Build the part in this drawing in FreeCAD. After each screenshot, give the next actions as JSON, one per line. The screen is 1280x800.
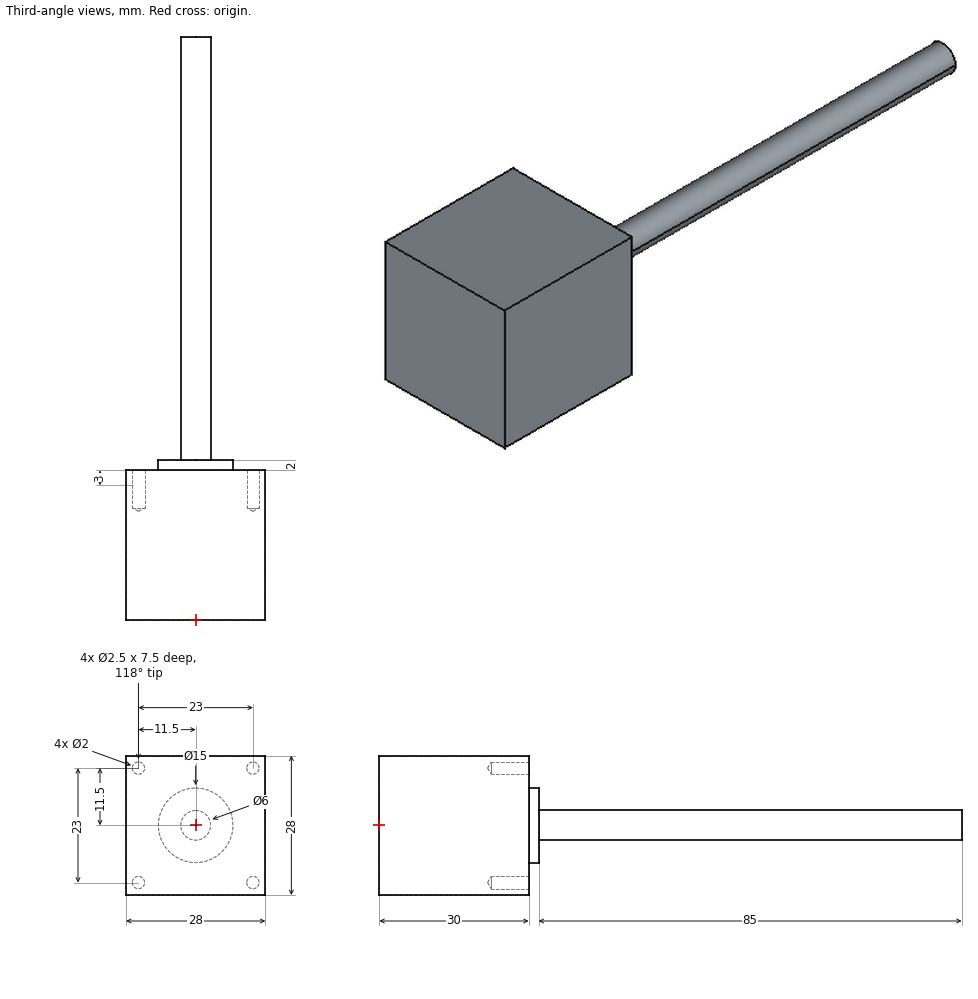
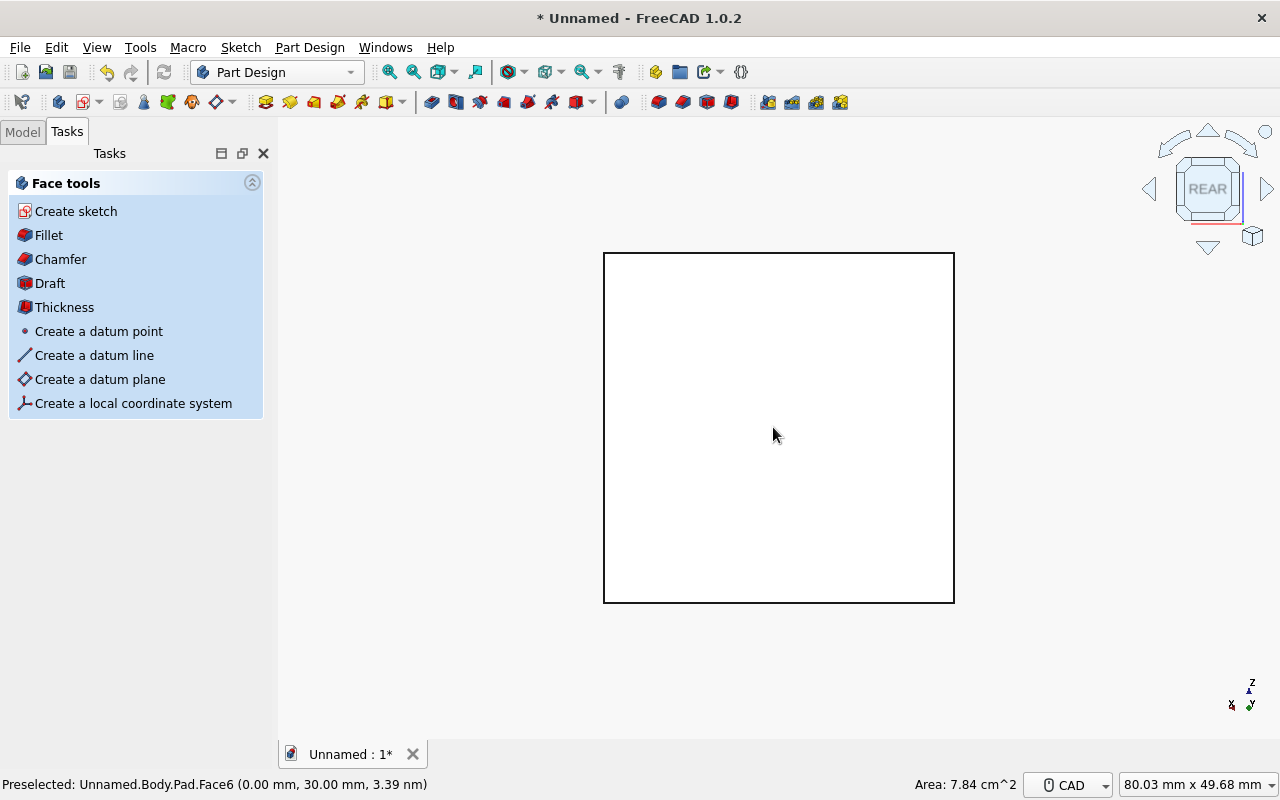
{"action": "left_click", "coordinate": [84, 102]}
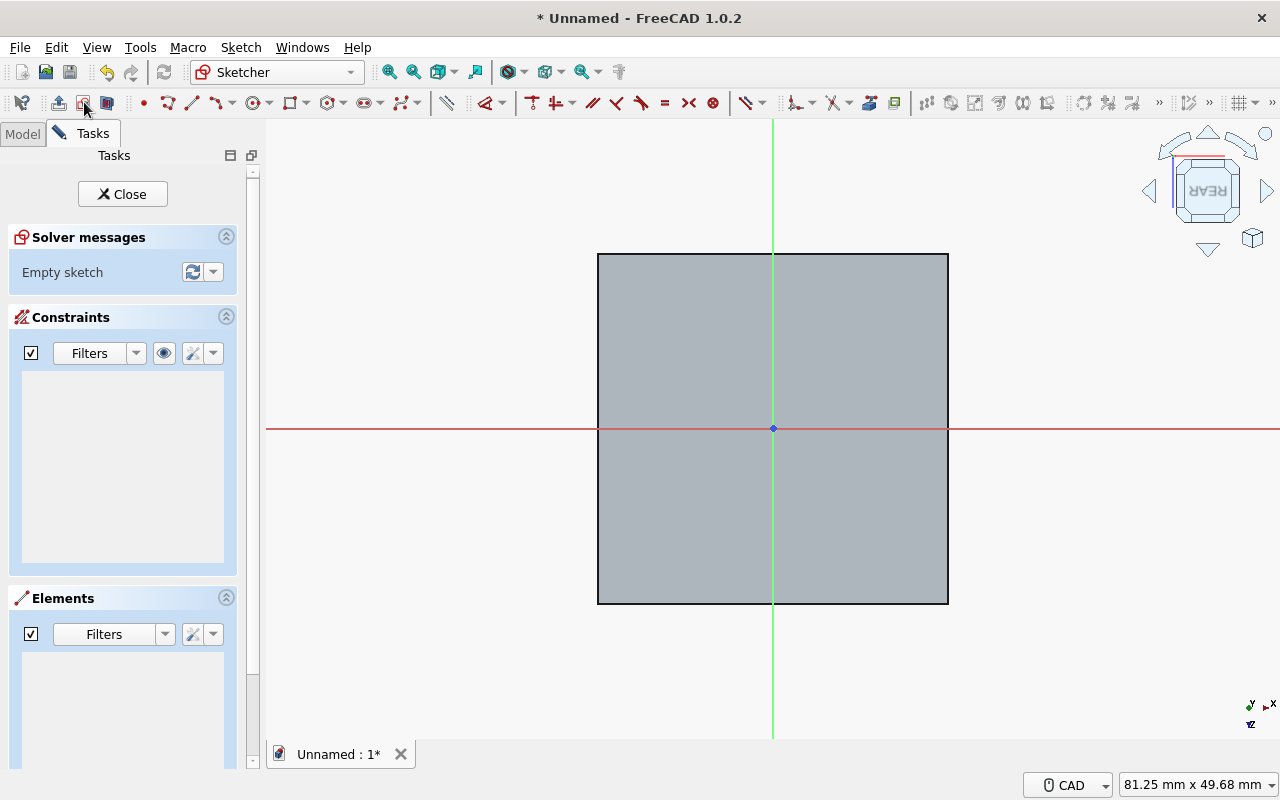
{"action": "scroll", "coordinate": [829, 429], "scroll_direction": "up", "scroll_amount": 4}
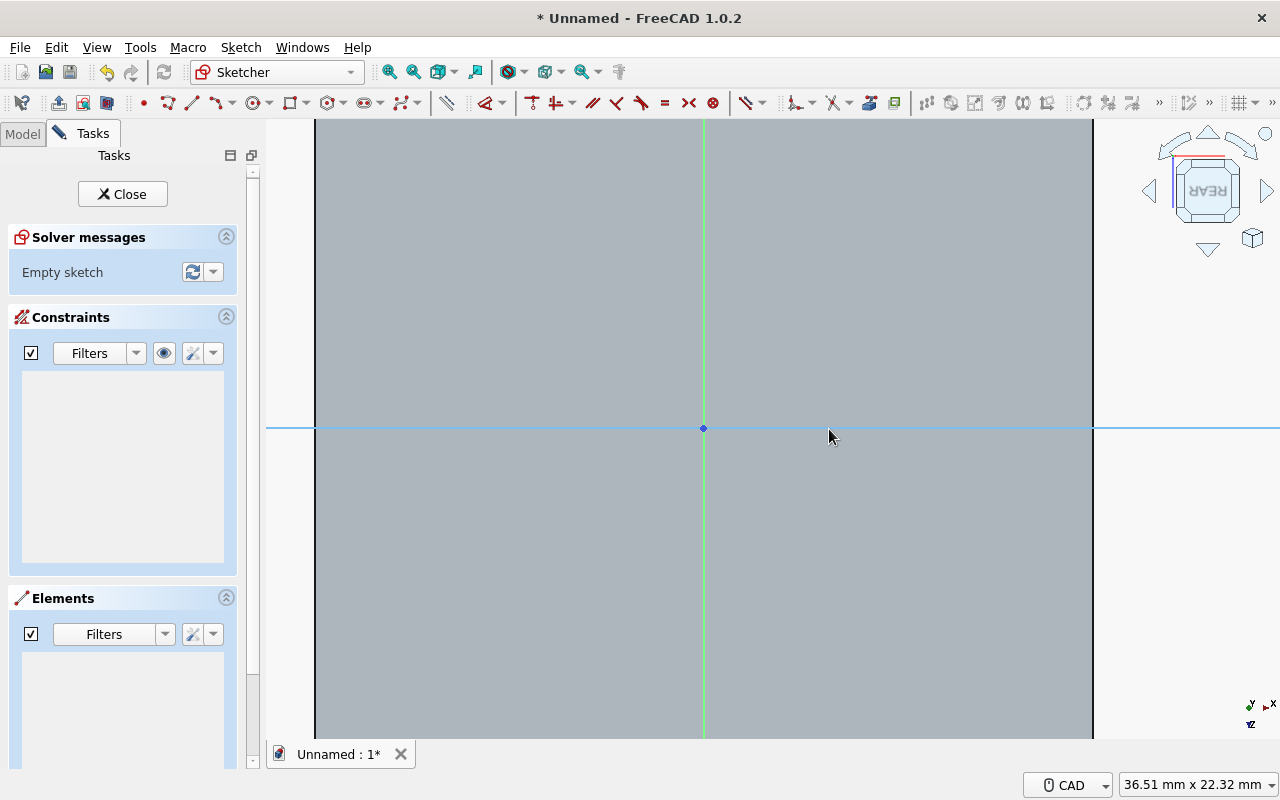
{"action": "left_click", "coordinate": [254, 104]}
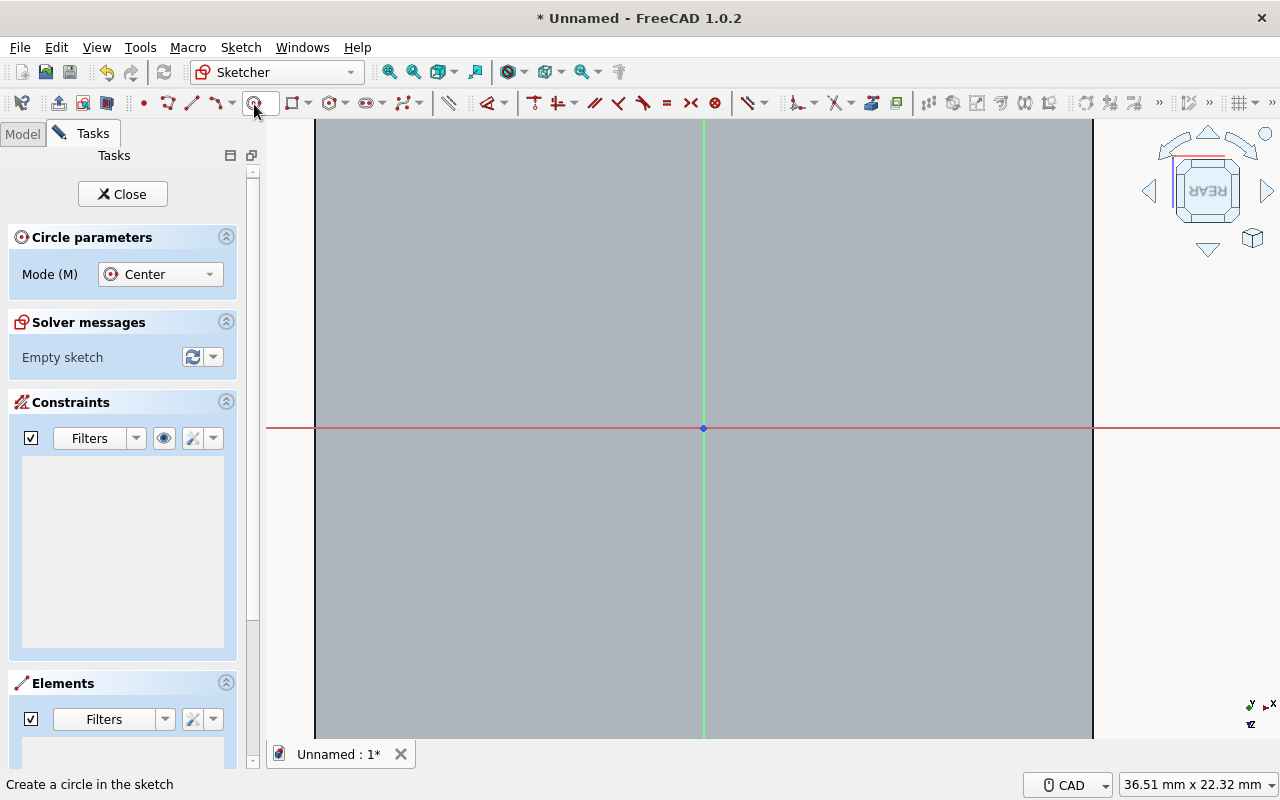
{"action": "left_click", "coordinate": [704, 428]}
{"action": "left_click", "coordinate": [851, 281]}
{"action": "key", "text": "Escape"}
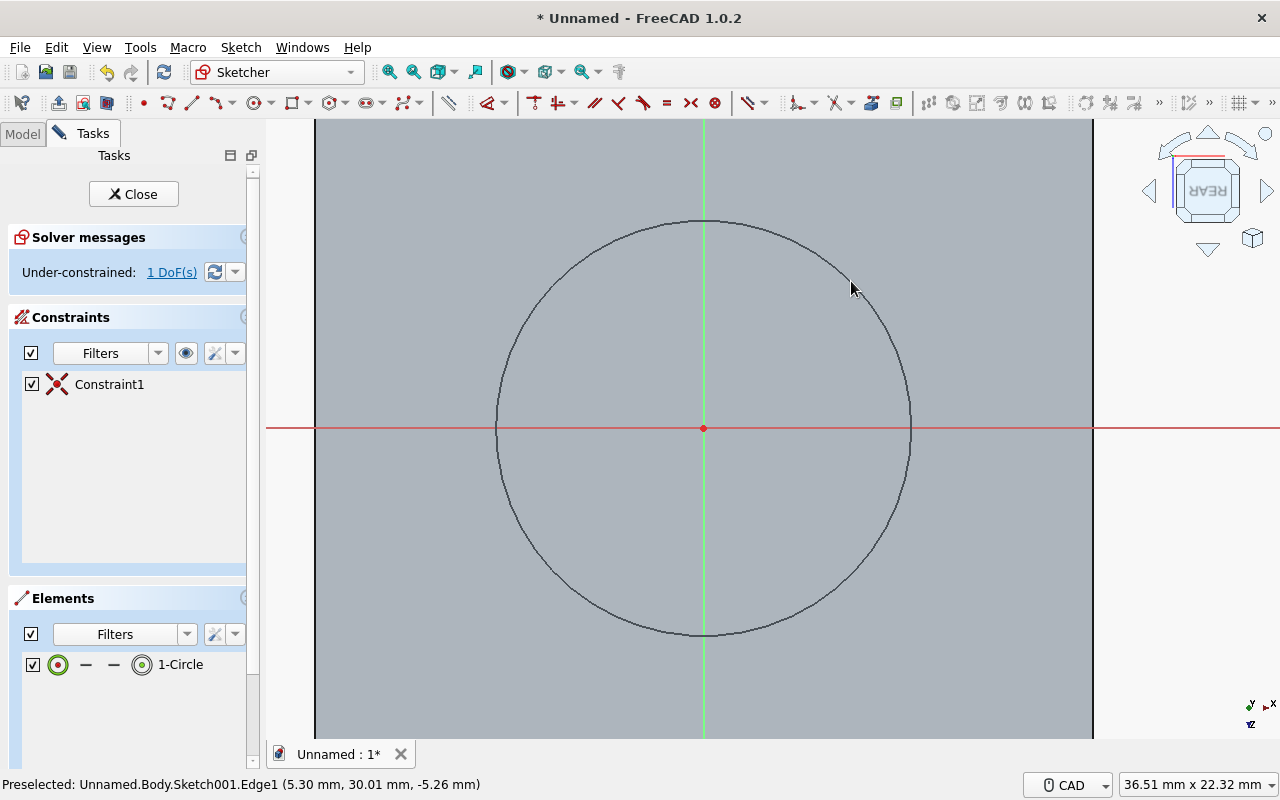
{"action": "left_click", "coordinate": [488, 104]}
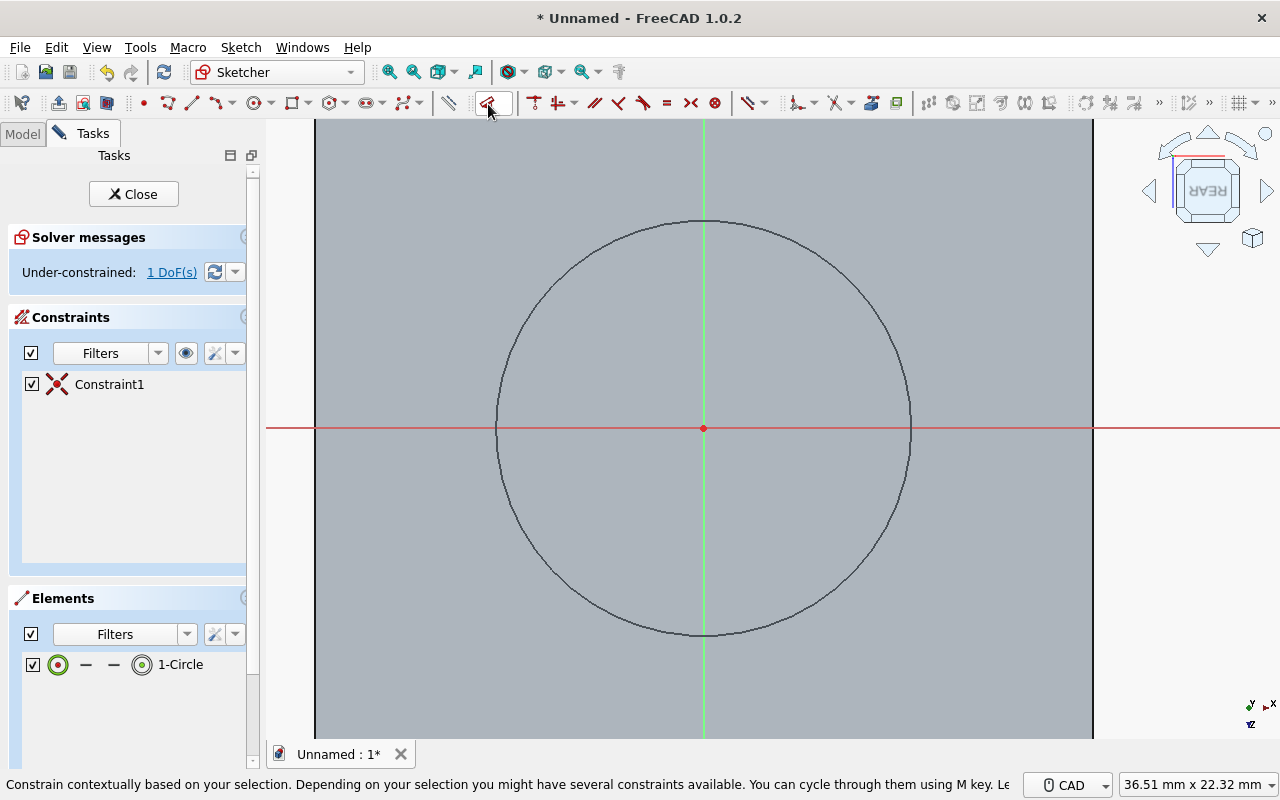
{"action": "left_click", "coordinate": [850, 281]}
{"action": "left_click", "coordinate": [873, 258]}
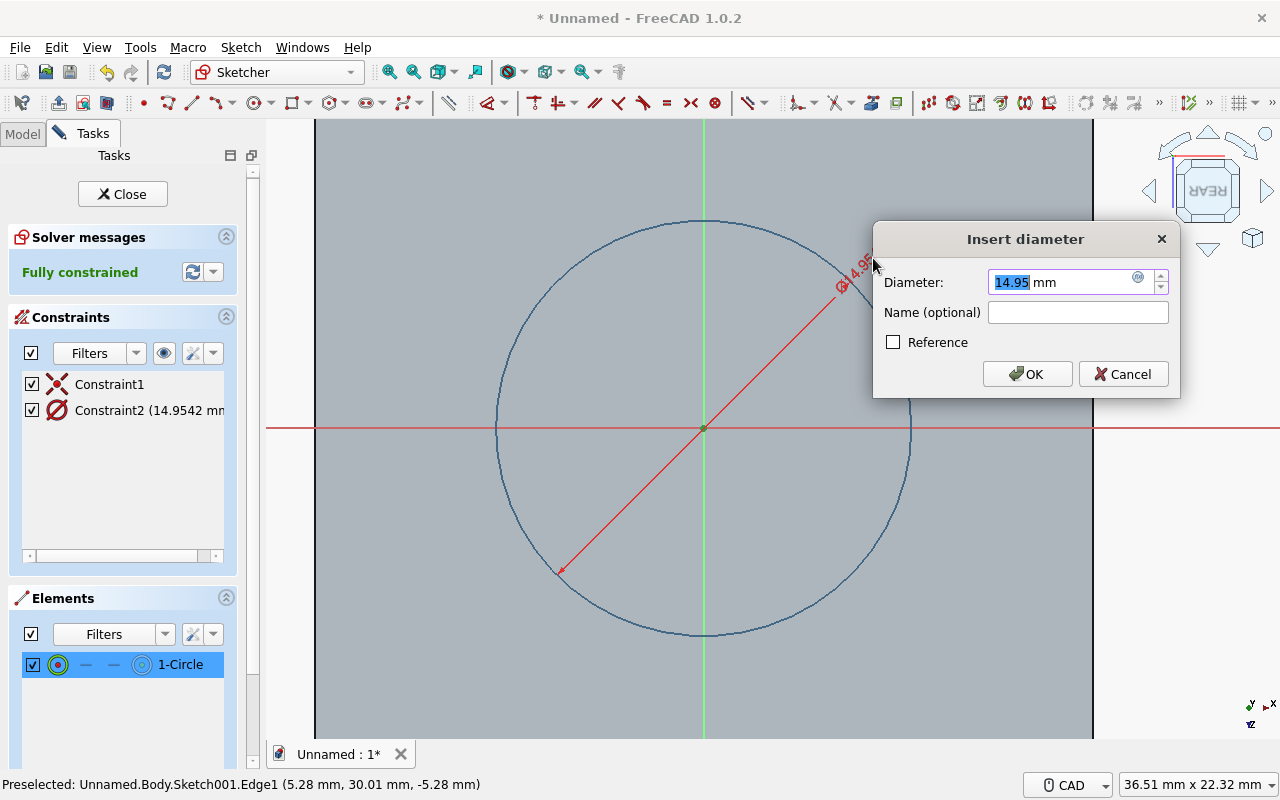
{"action": "type", "text": "15"}
{"action": "key", "text": "Return"}
{"action": "key", "text": "Escape"}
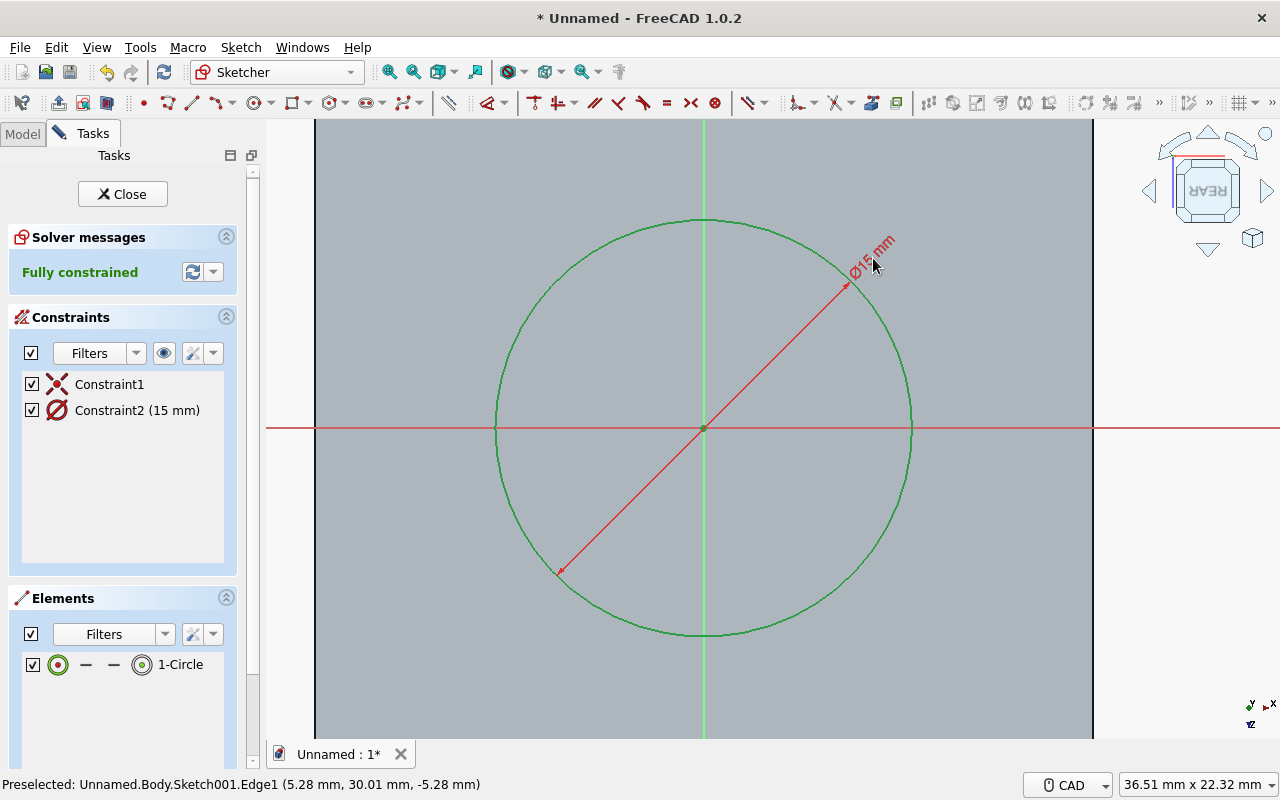
{"action": "left_click", "coordinate": [123, 194]}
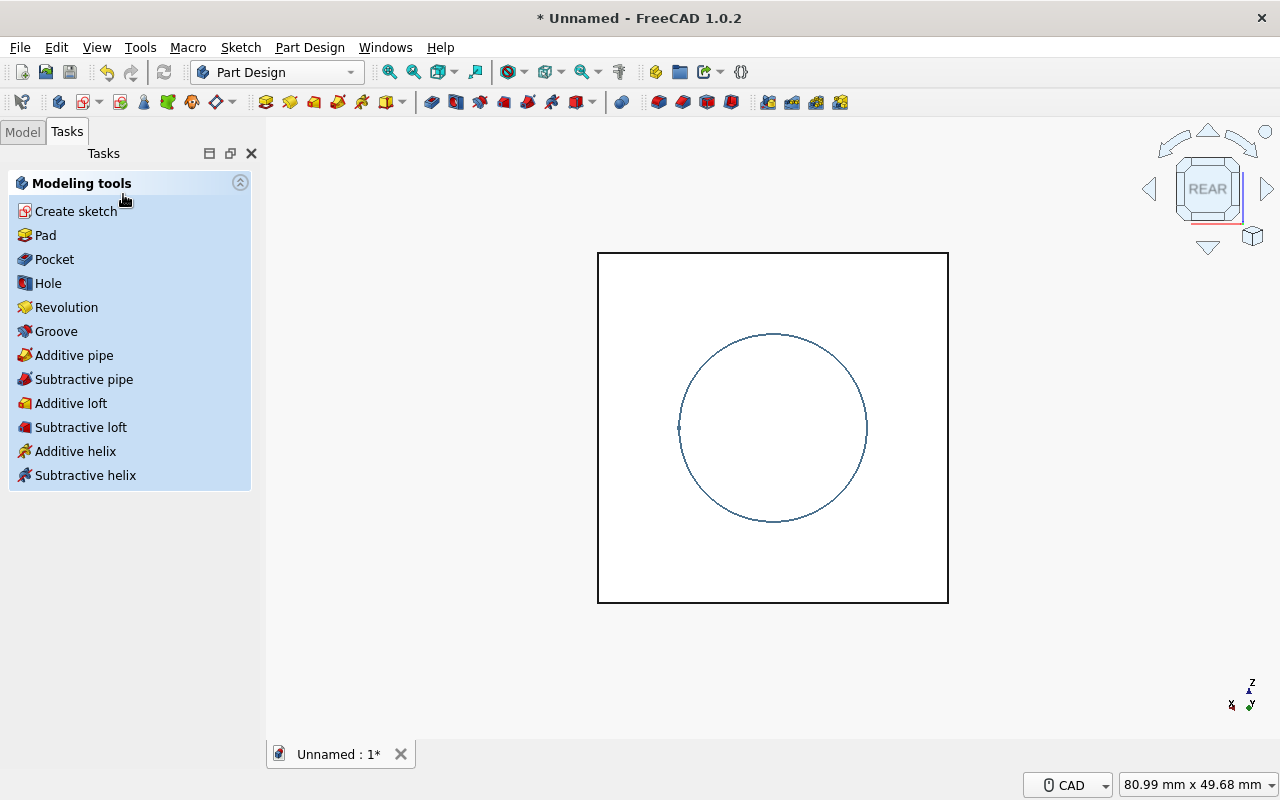
{"action": "left_click", "coordinate": [266, 102]}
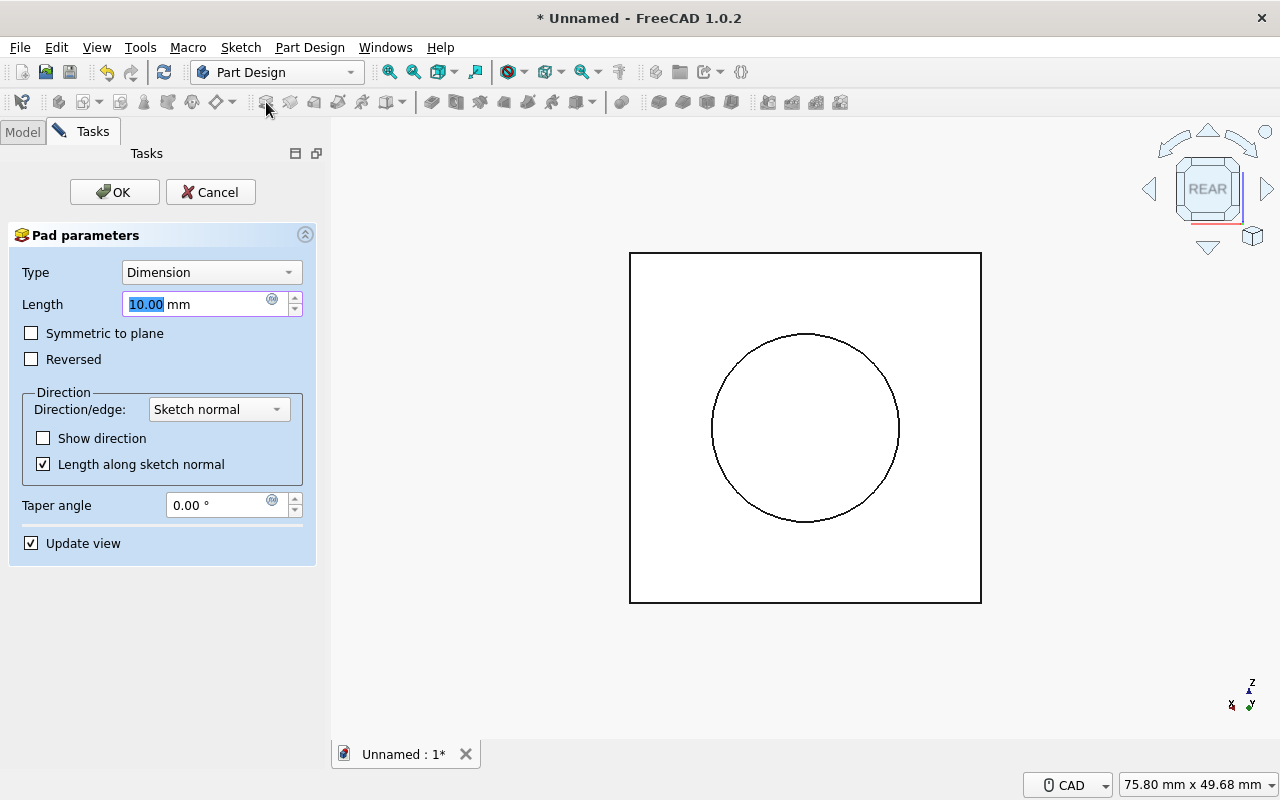
{"action": "type", "text": "2"}
{"action": "key", "text": "Tab"}